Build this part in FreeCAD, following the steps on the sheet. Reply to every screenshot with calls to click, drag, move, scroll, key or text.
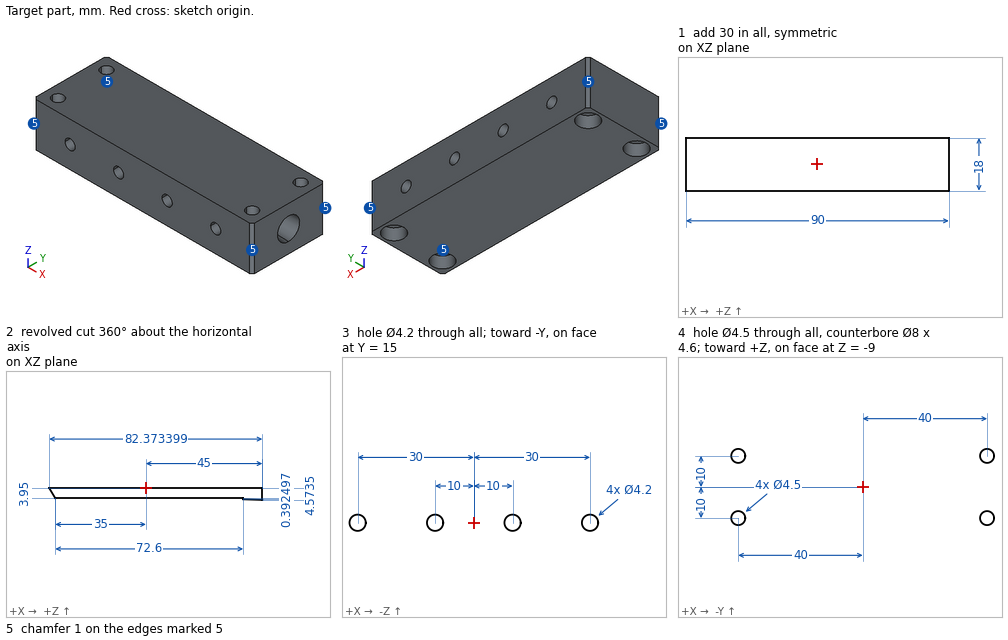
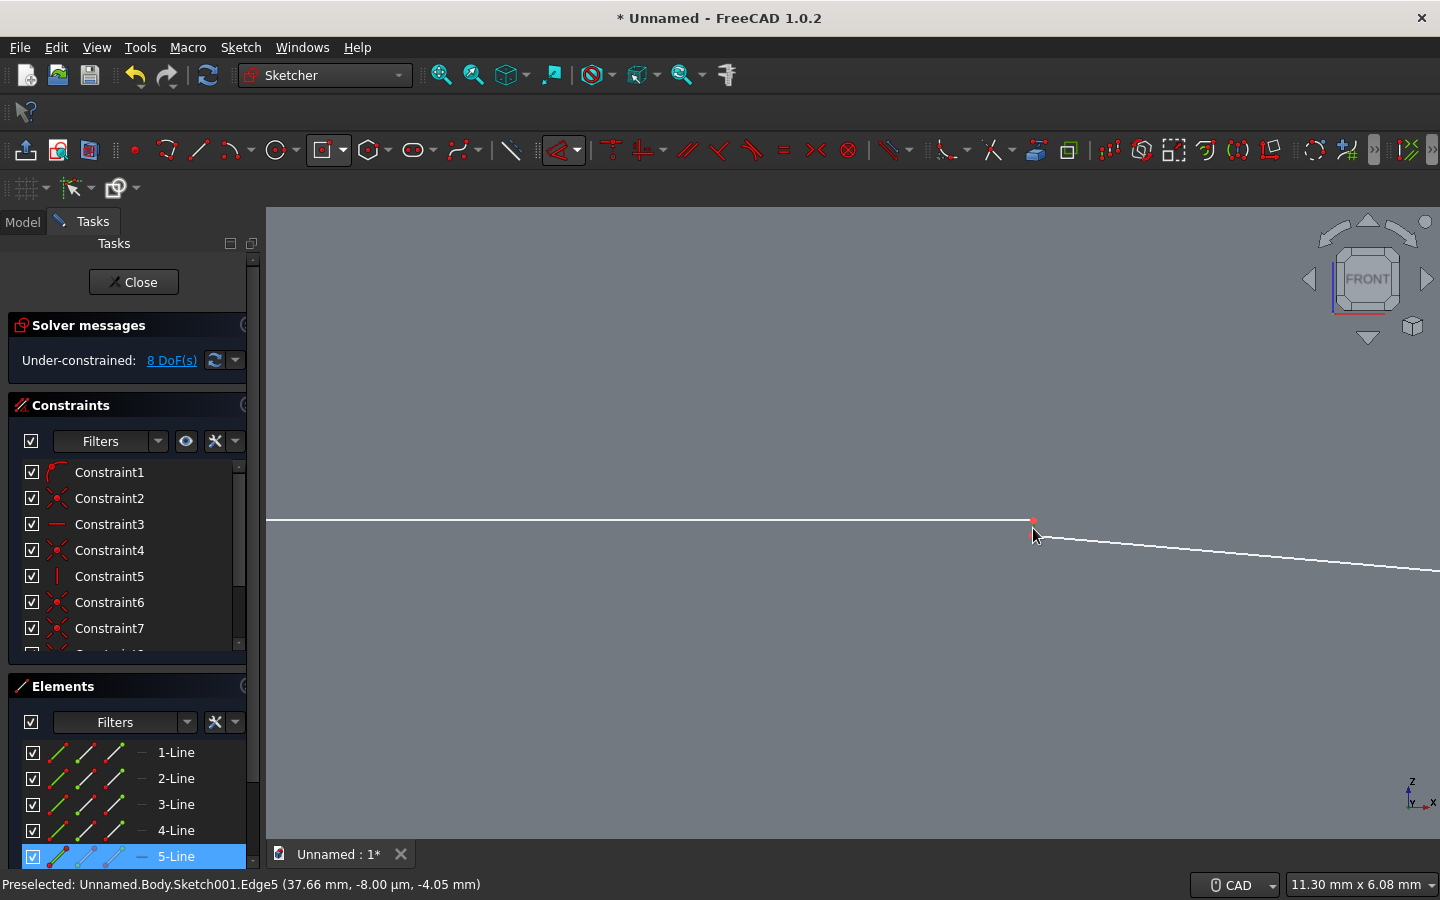
click(666, 150)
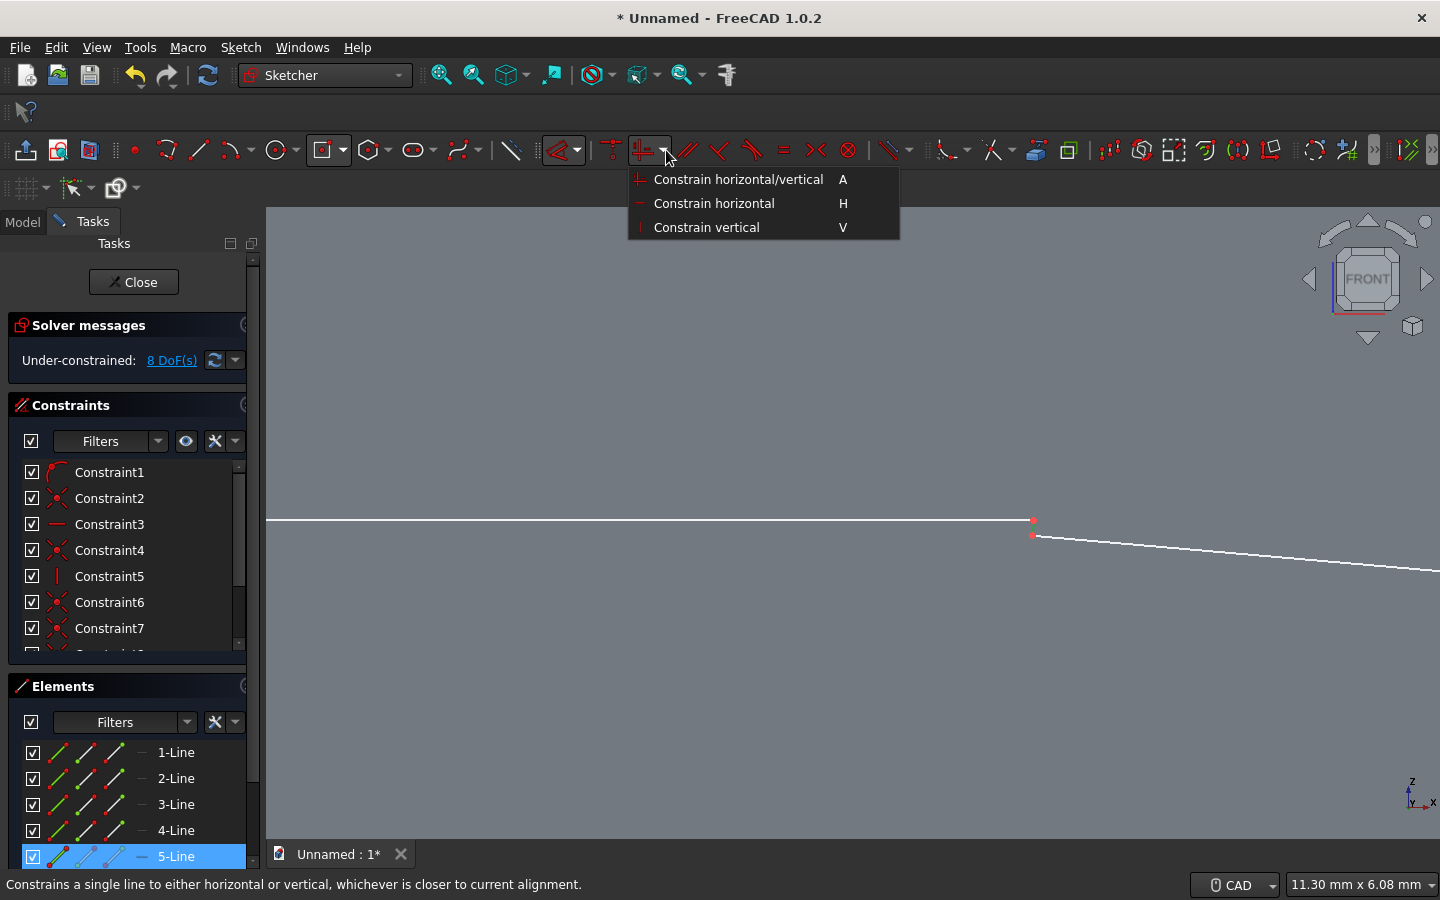
click(764, 227)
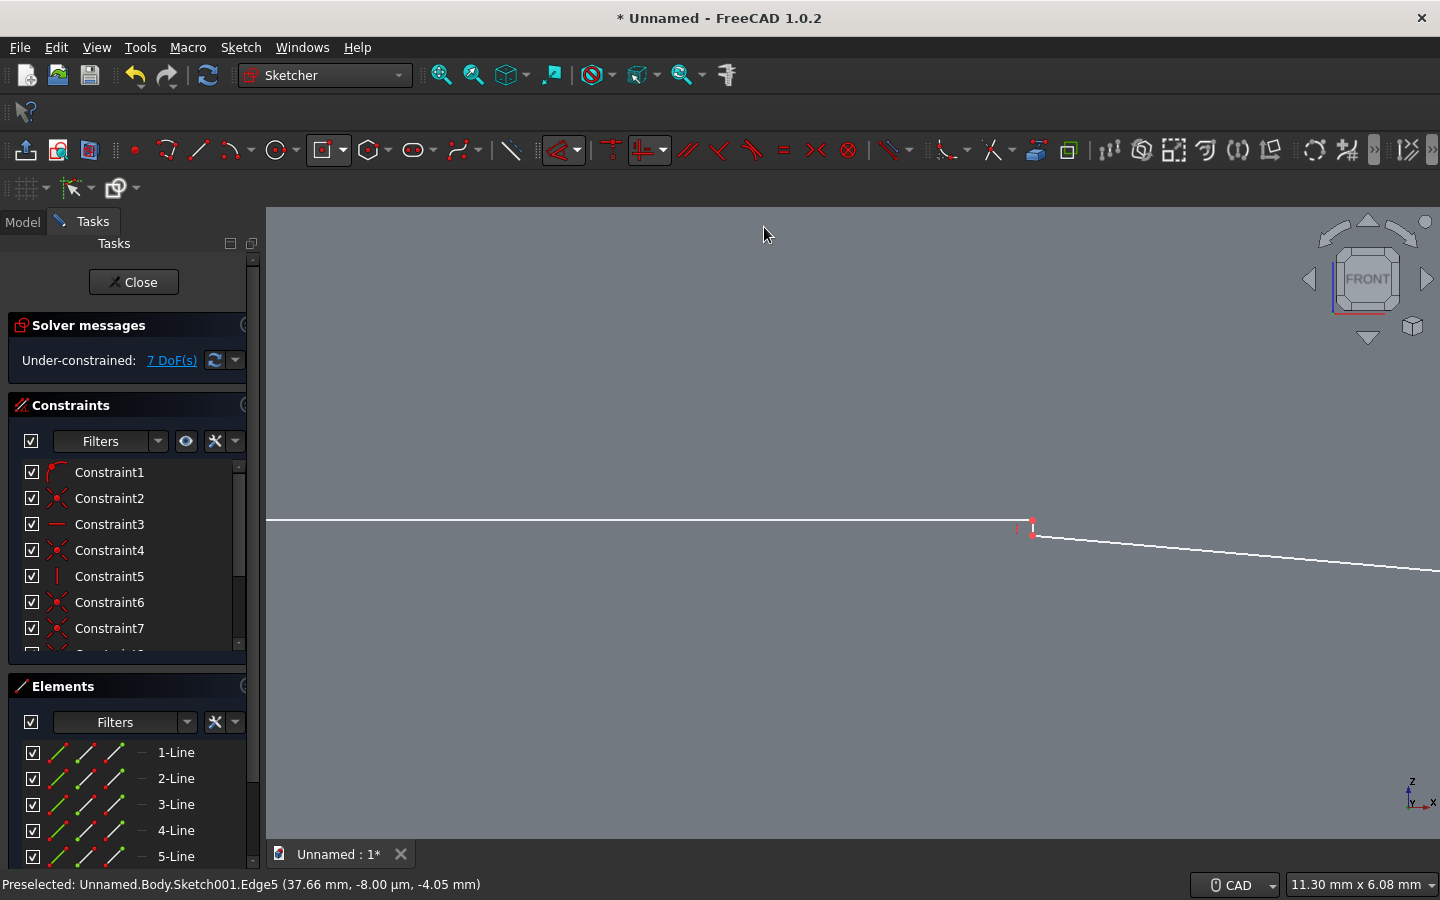
scroll(1047, 537, down, 13)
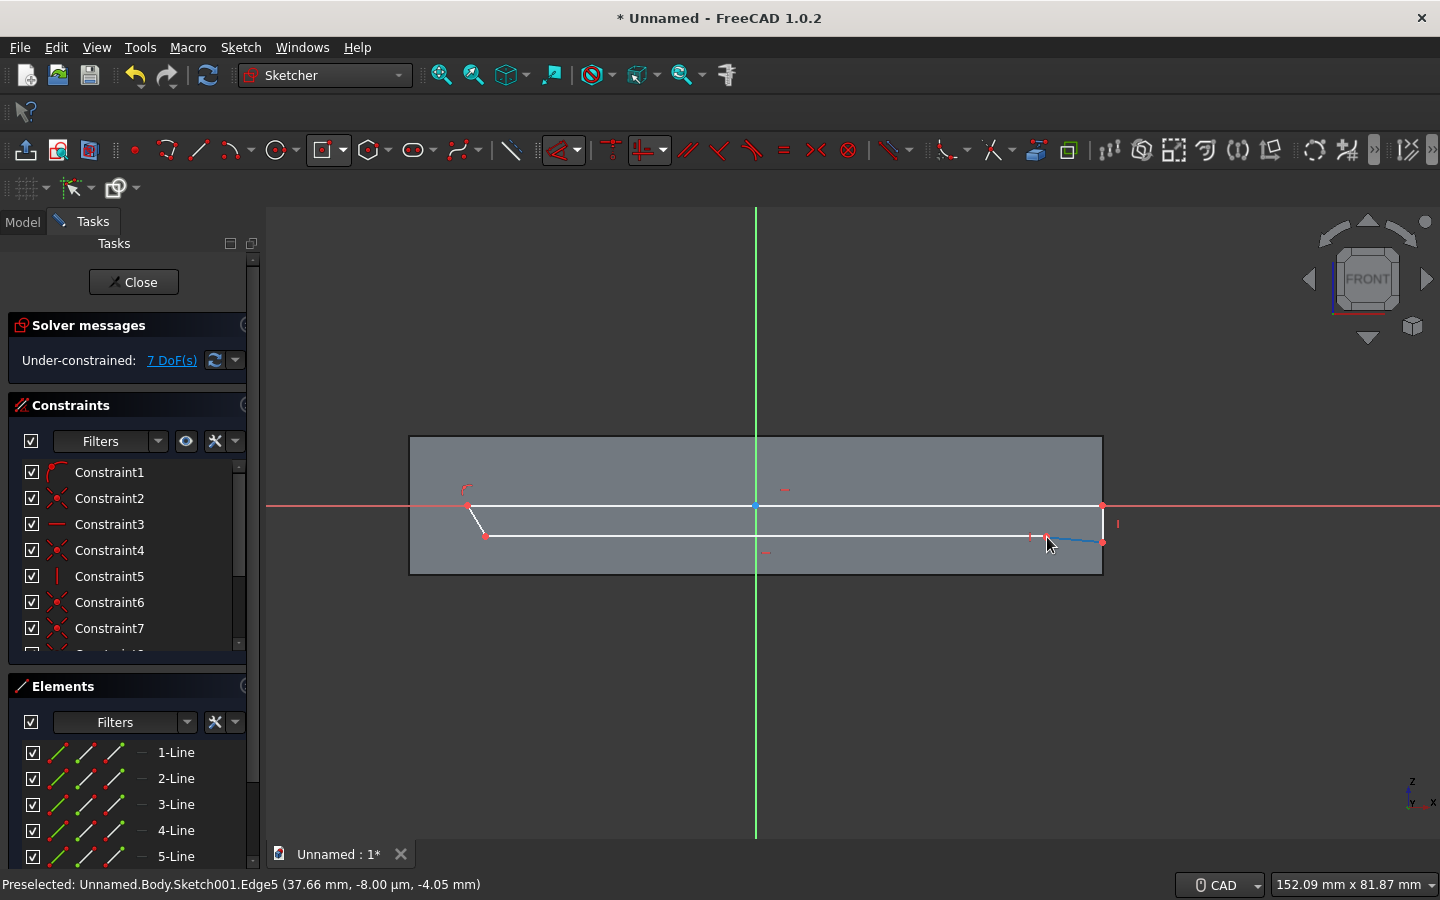
click(486, 536)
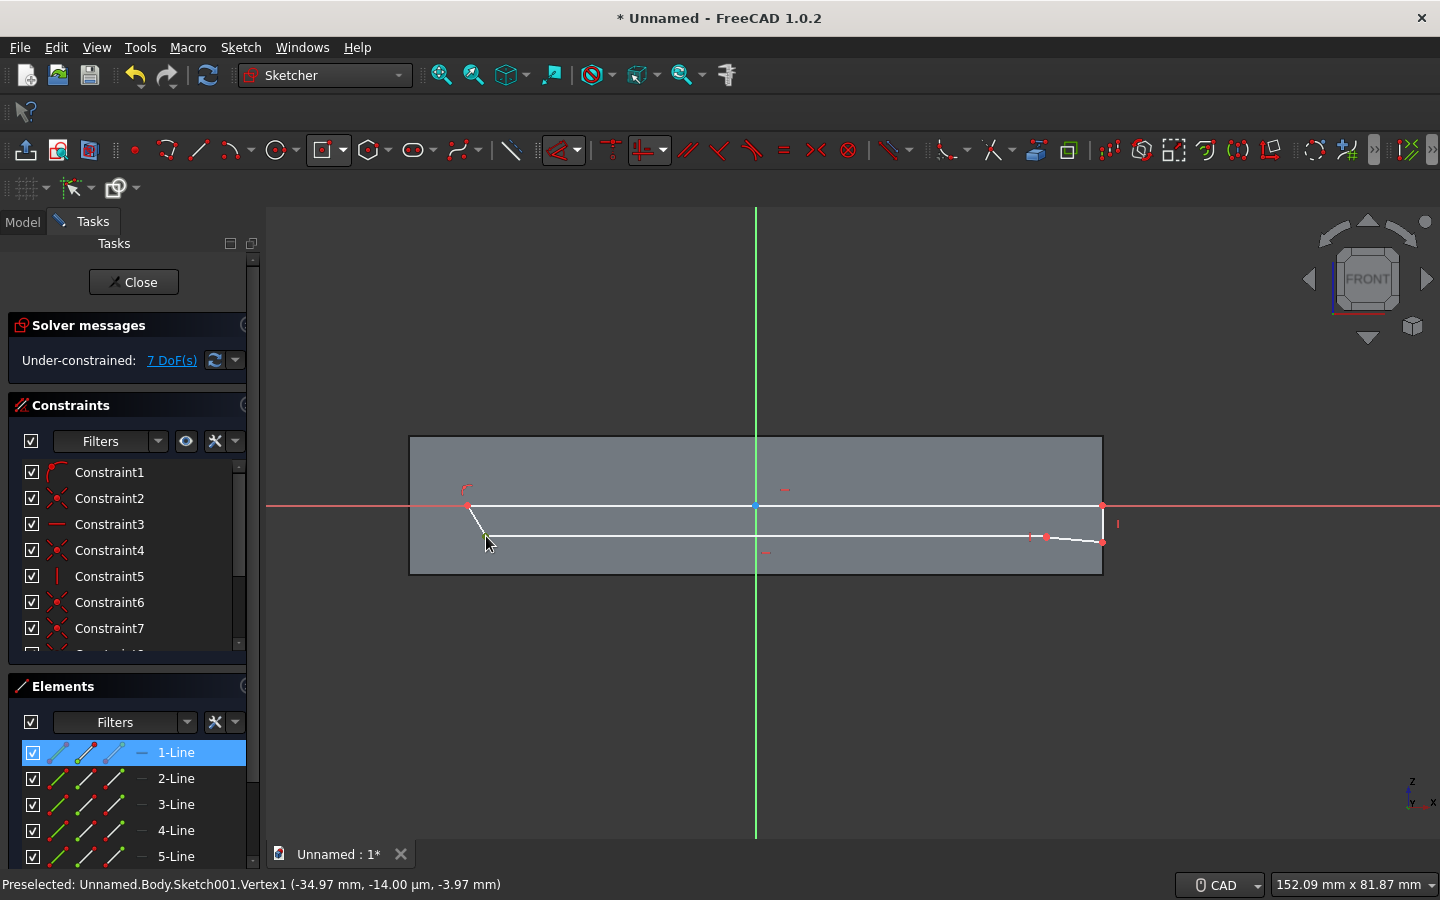
click(580, 150)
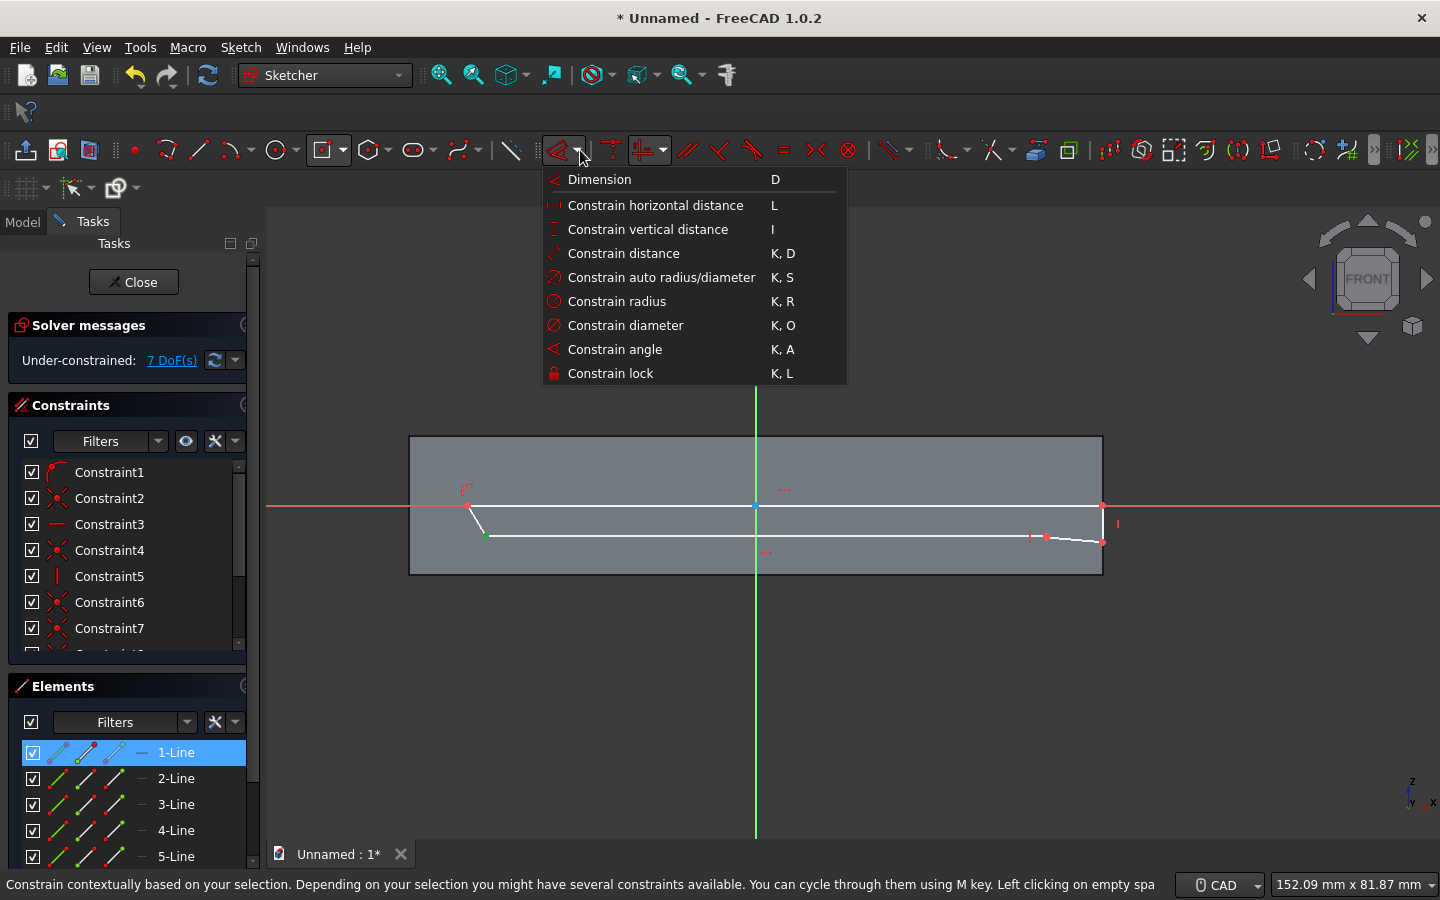
click(695, 205)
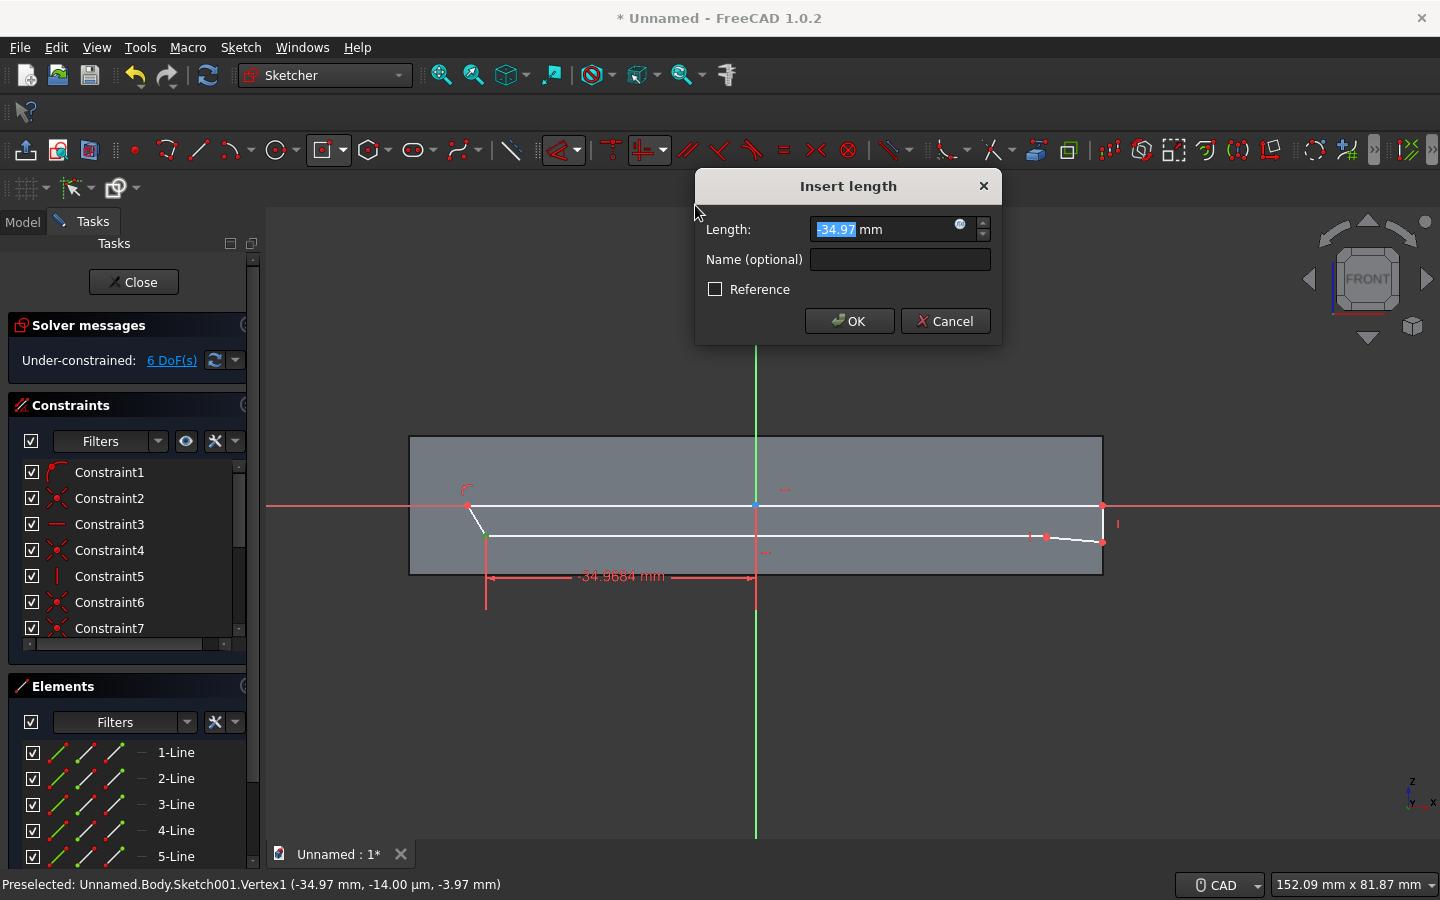
text(-35)
key(Return)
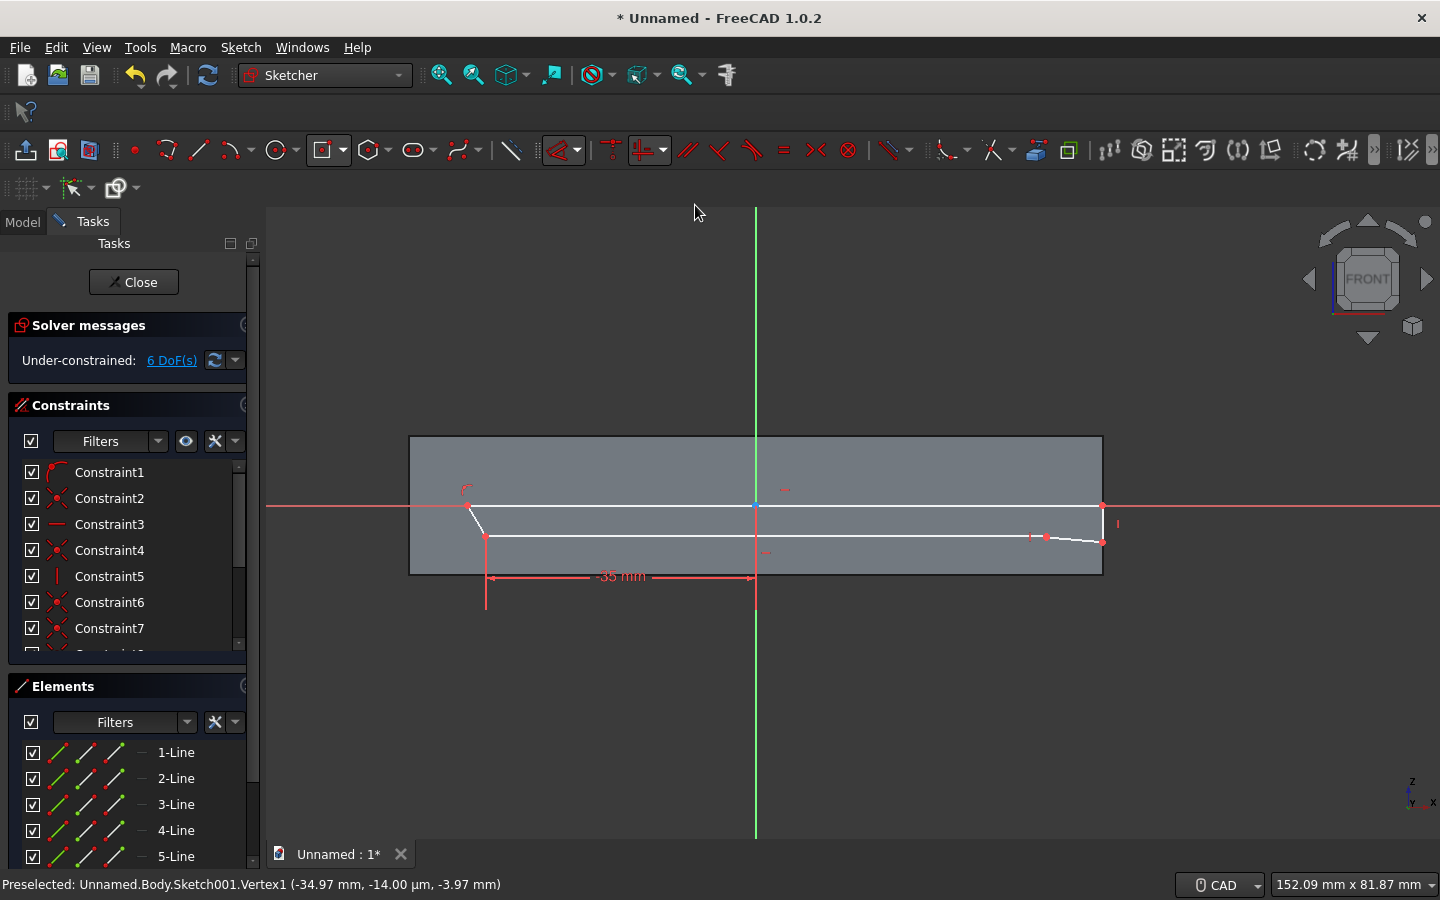
click(1103, 506)